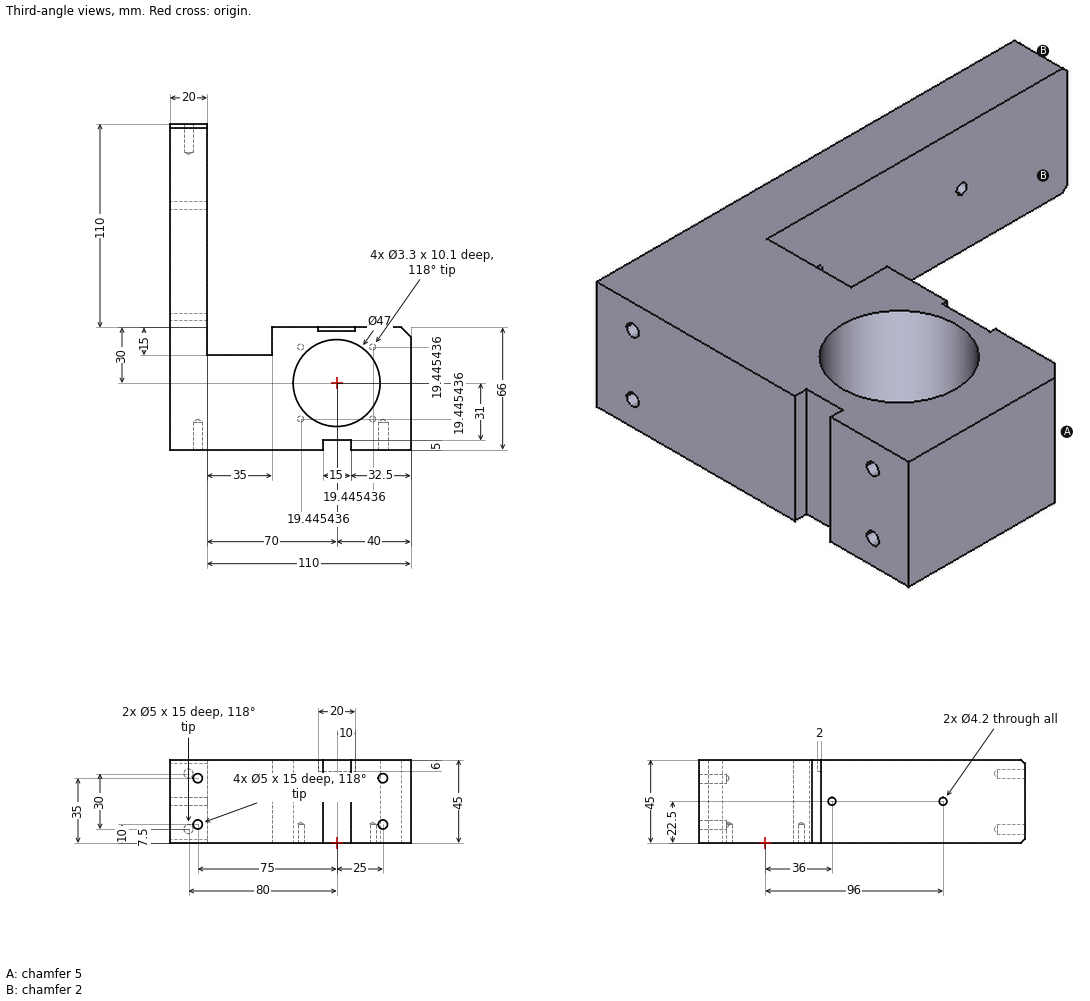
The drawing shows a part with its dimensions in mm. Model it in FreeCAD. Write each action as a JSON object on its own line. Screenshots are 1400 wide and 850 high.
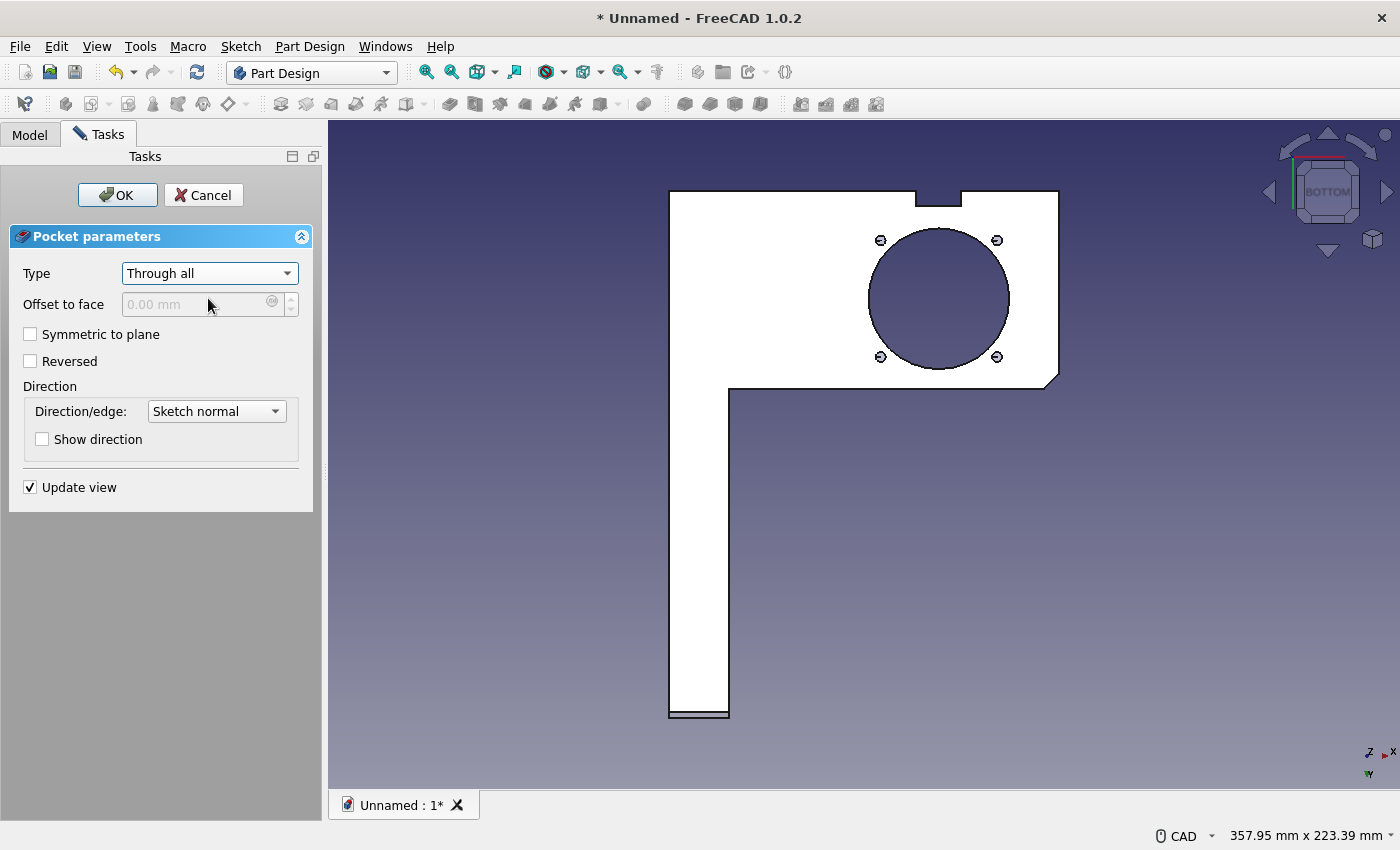
{"action": "left_click", "coordinate": [31, 361]}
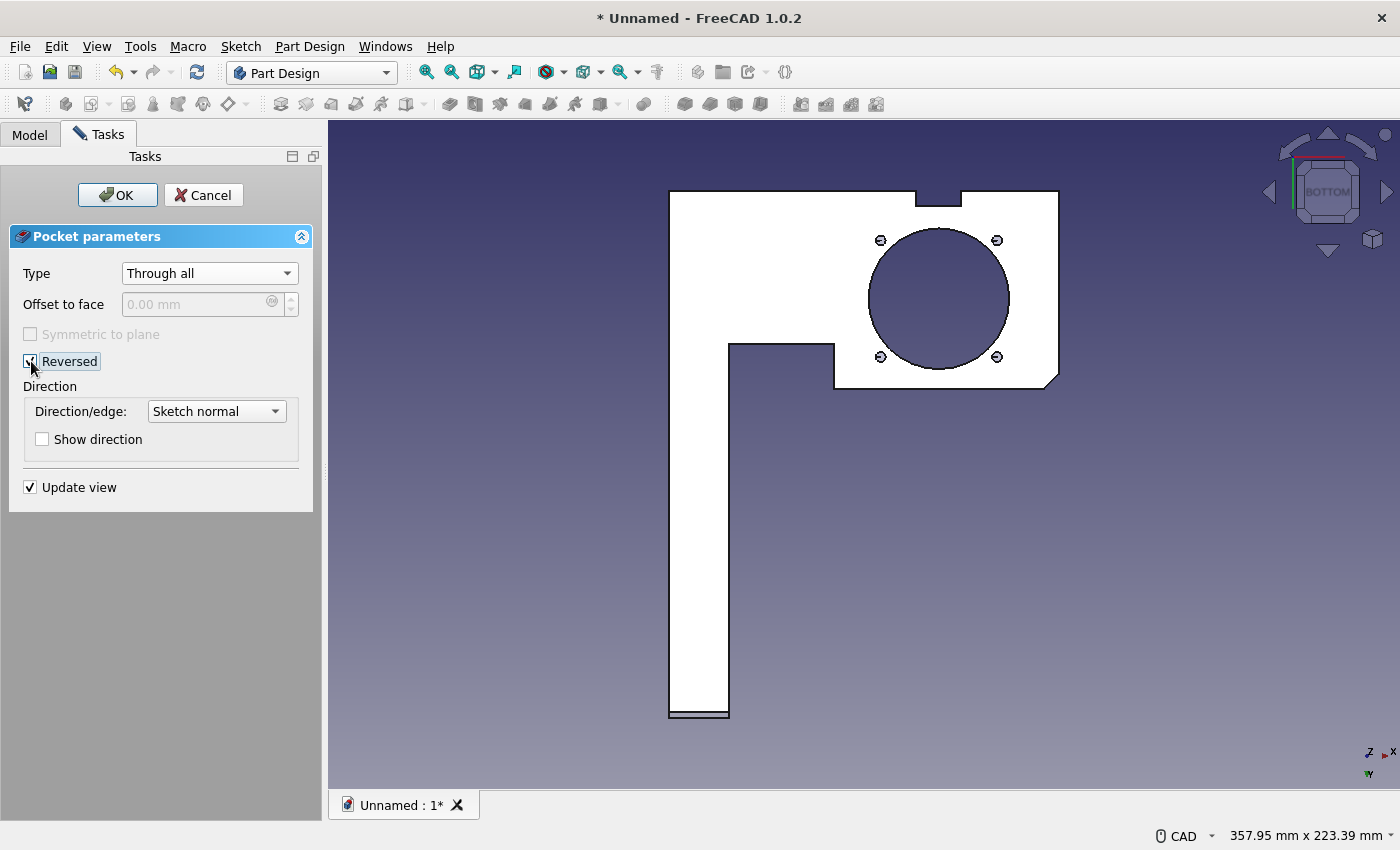
{"action": "left_click", "coordinate": [118, 195]}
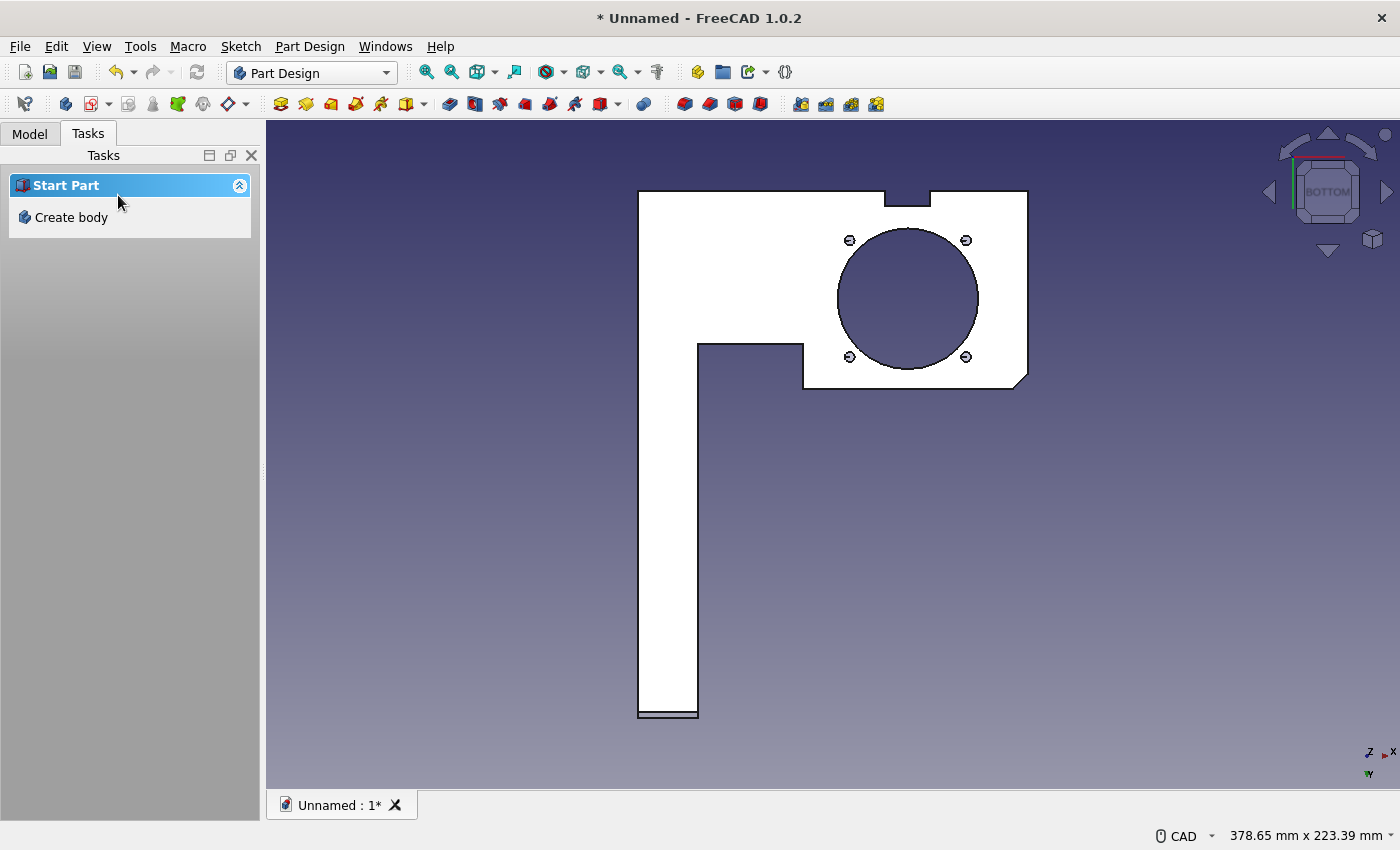
{"action": "key", "text": "4"}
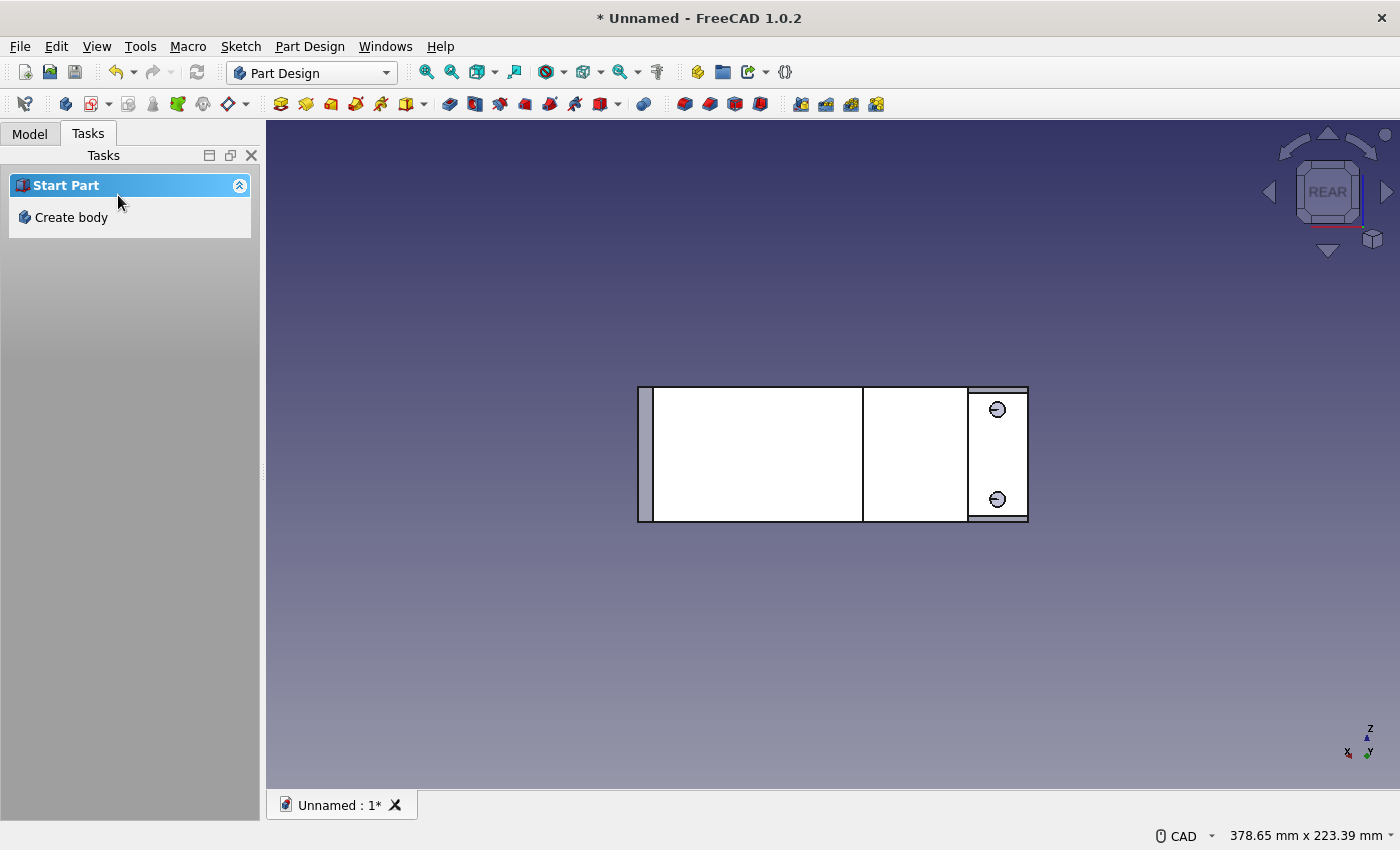
{"action": "left_click", "coordinate": [427, 72]}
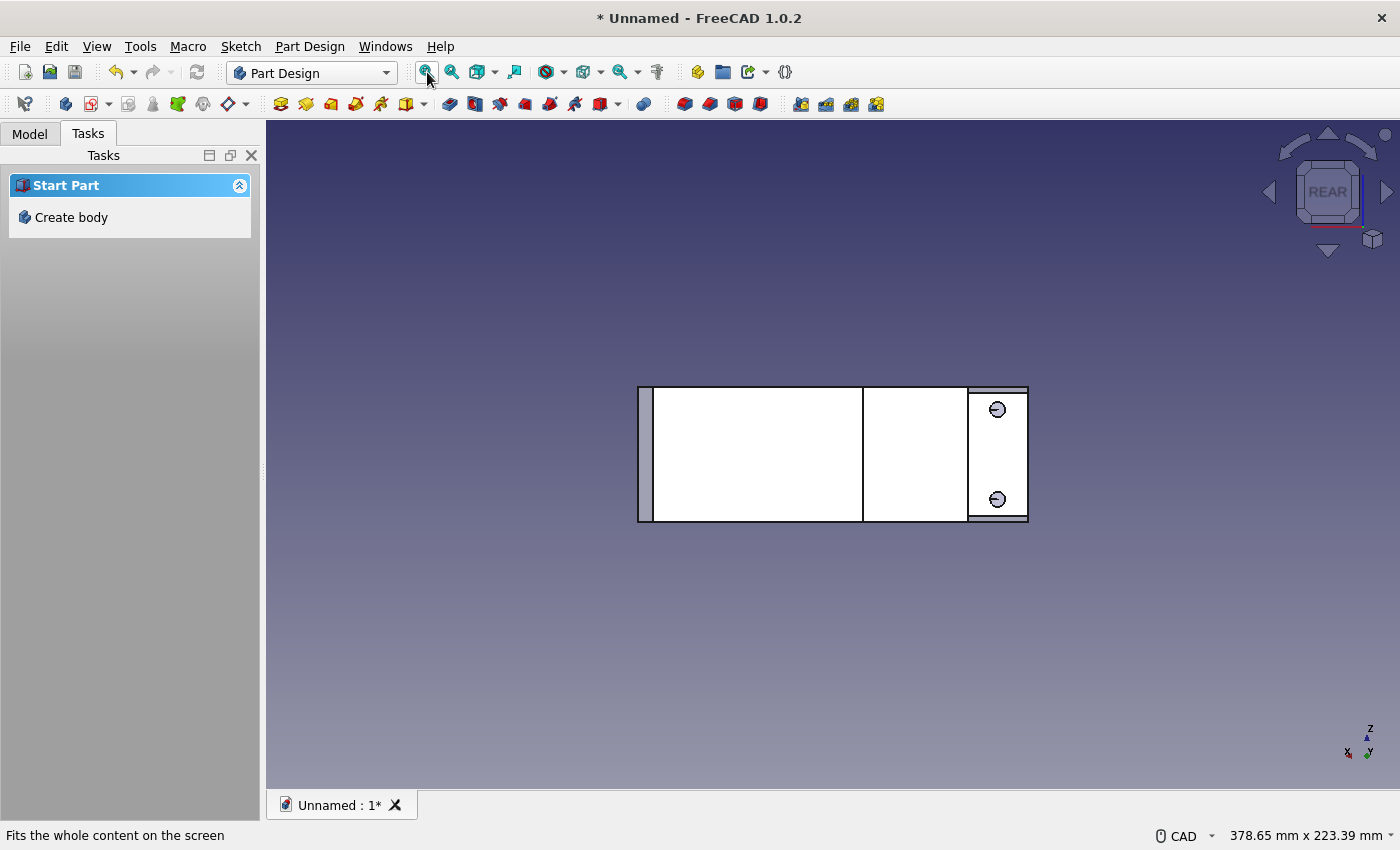
{"action": "left_click", "coordinate": [728, 454]}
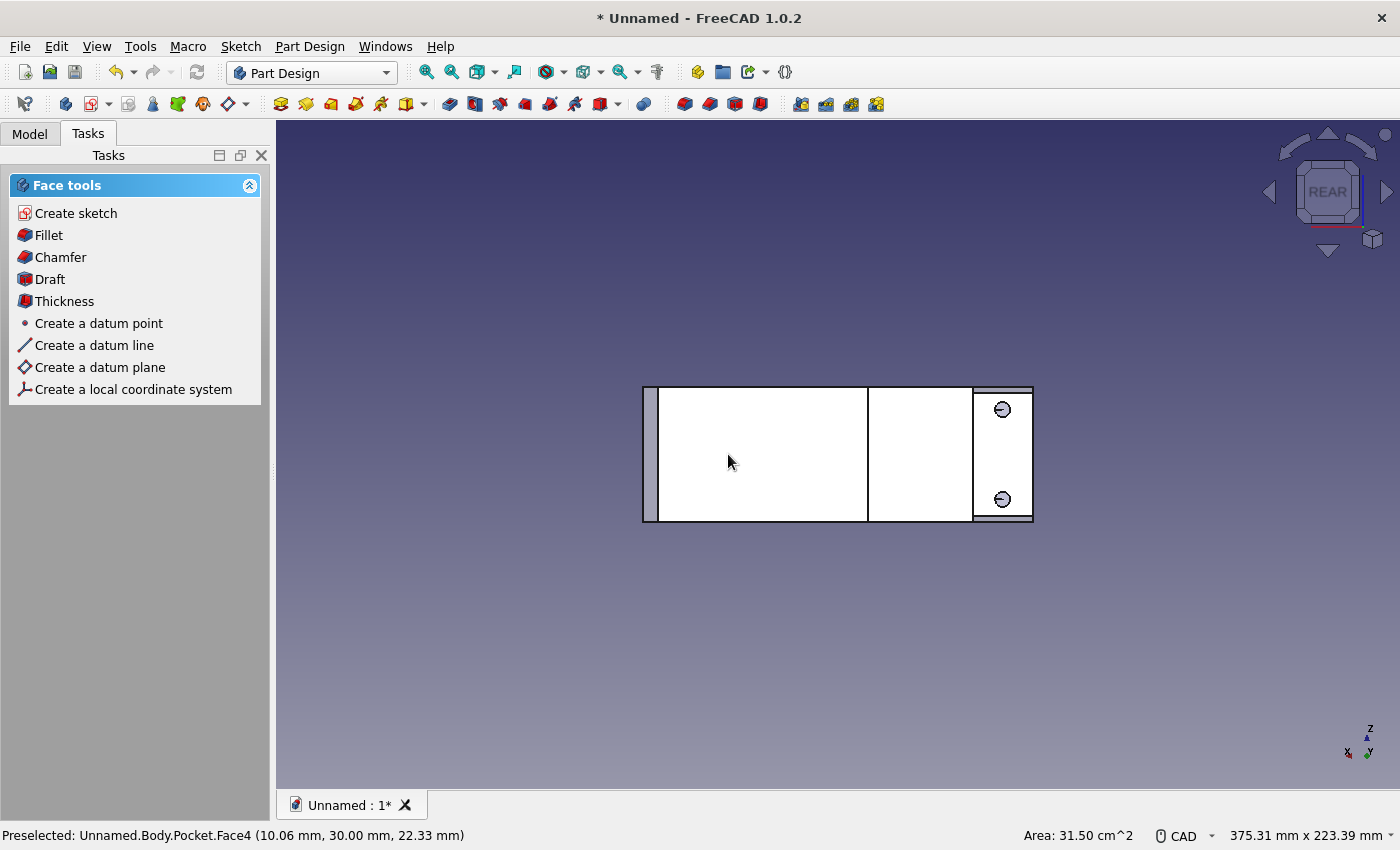
{"action": "left_click", "coordinate": [90, 104]}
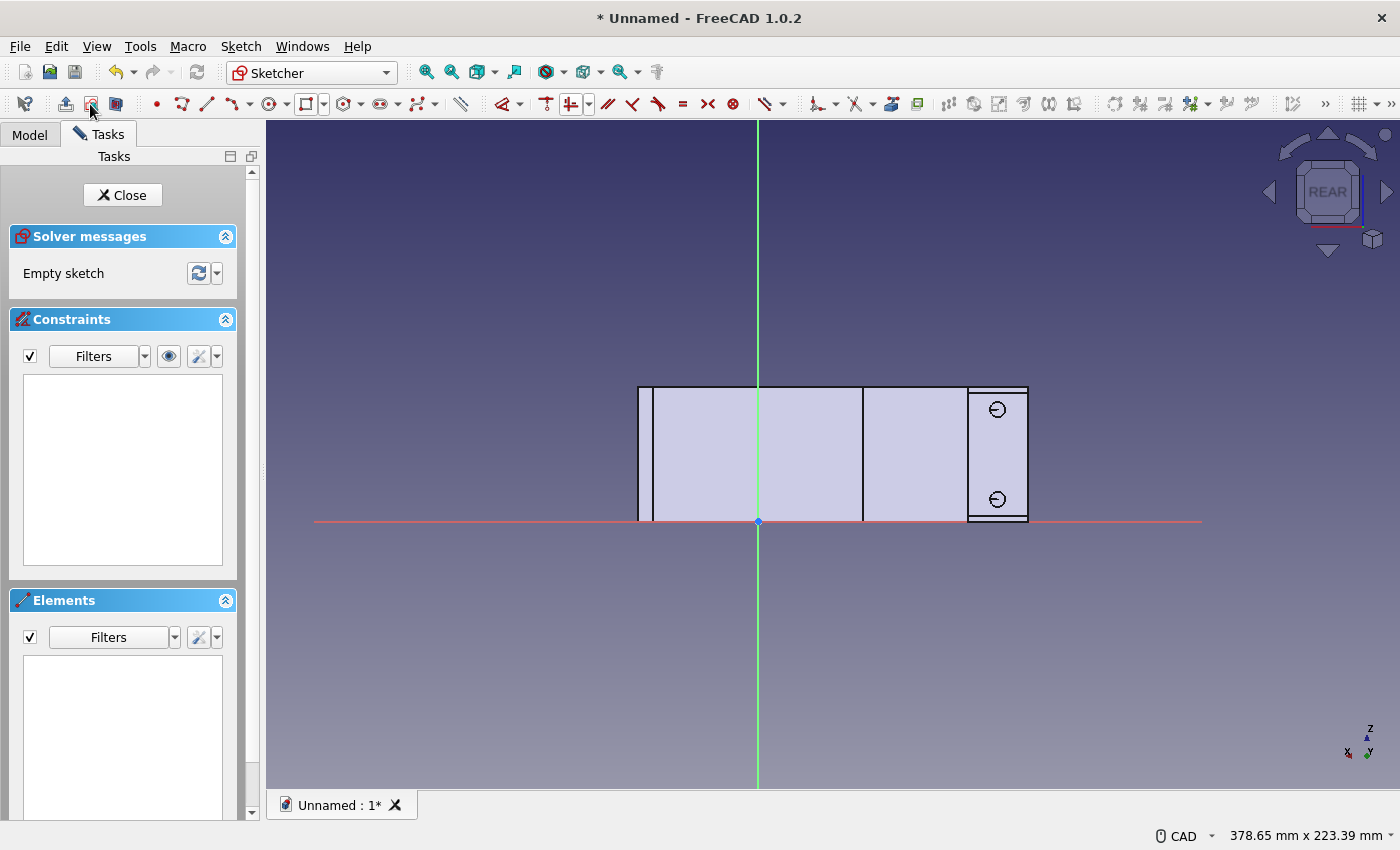
{"action": "left_click", "coordinate": [116, 104]}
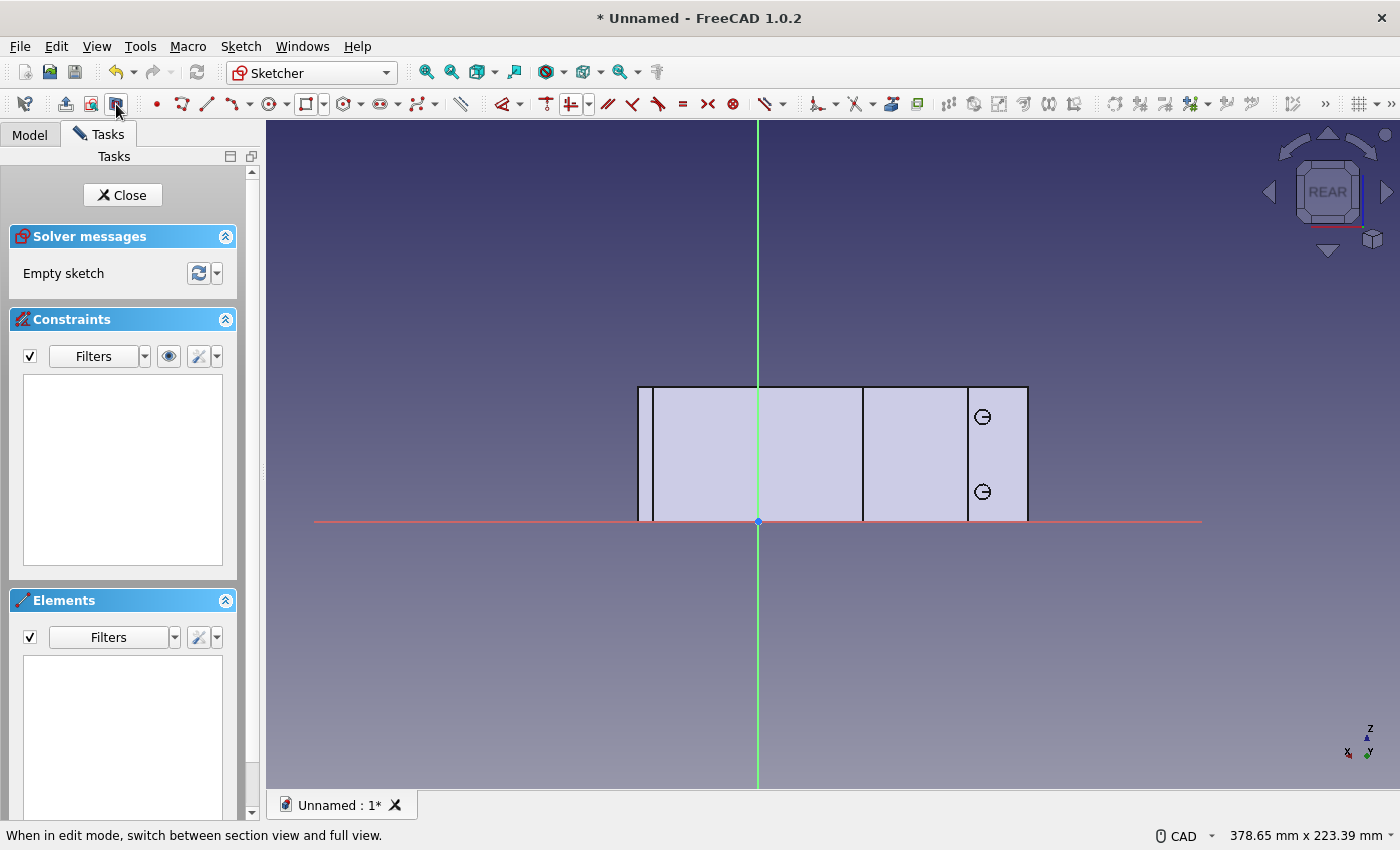
{"action": "scroll", "coordinate": [755, 455], "scroll_direction": "up", "scroll_amount": 6}